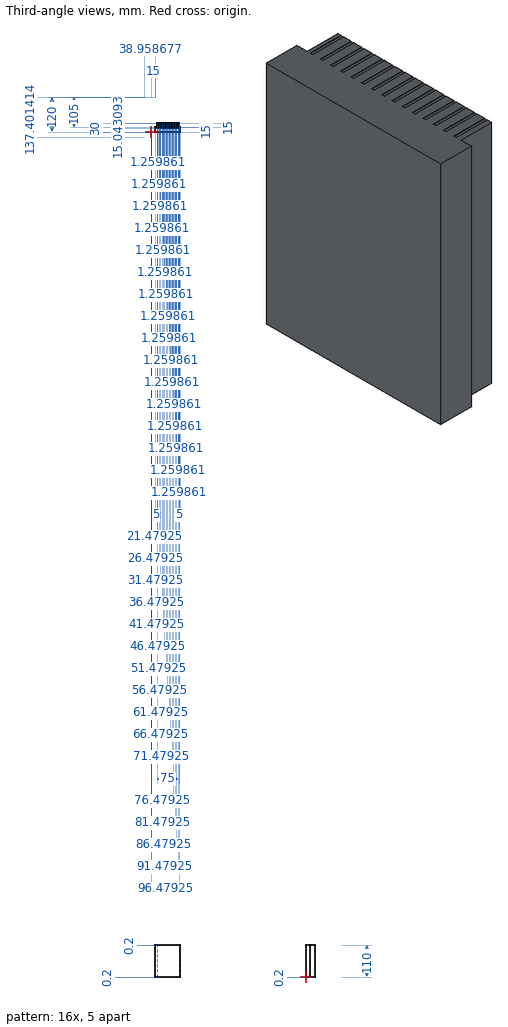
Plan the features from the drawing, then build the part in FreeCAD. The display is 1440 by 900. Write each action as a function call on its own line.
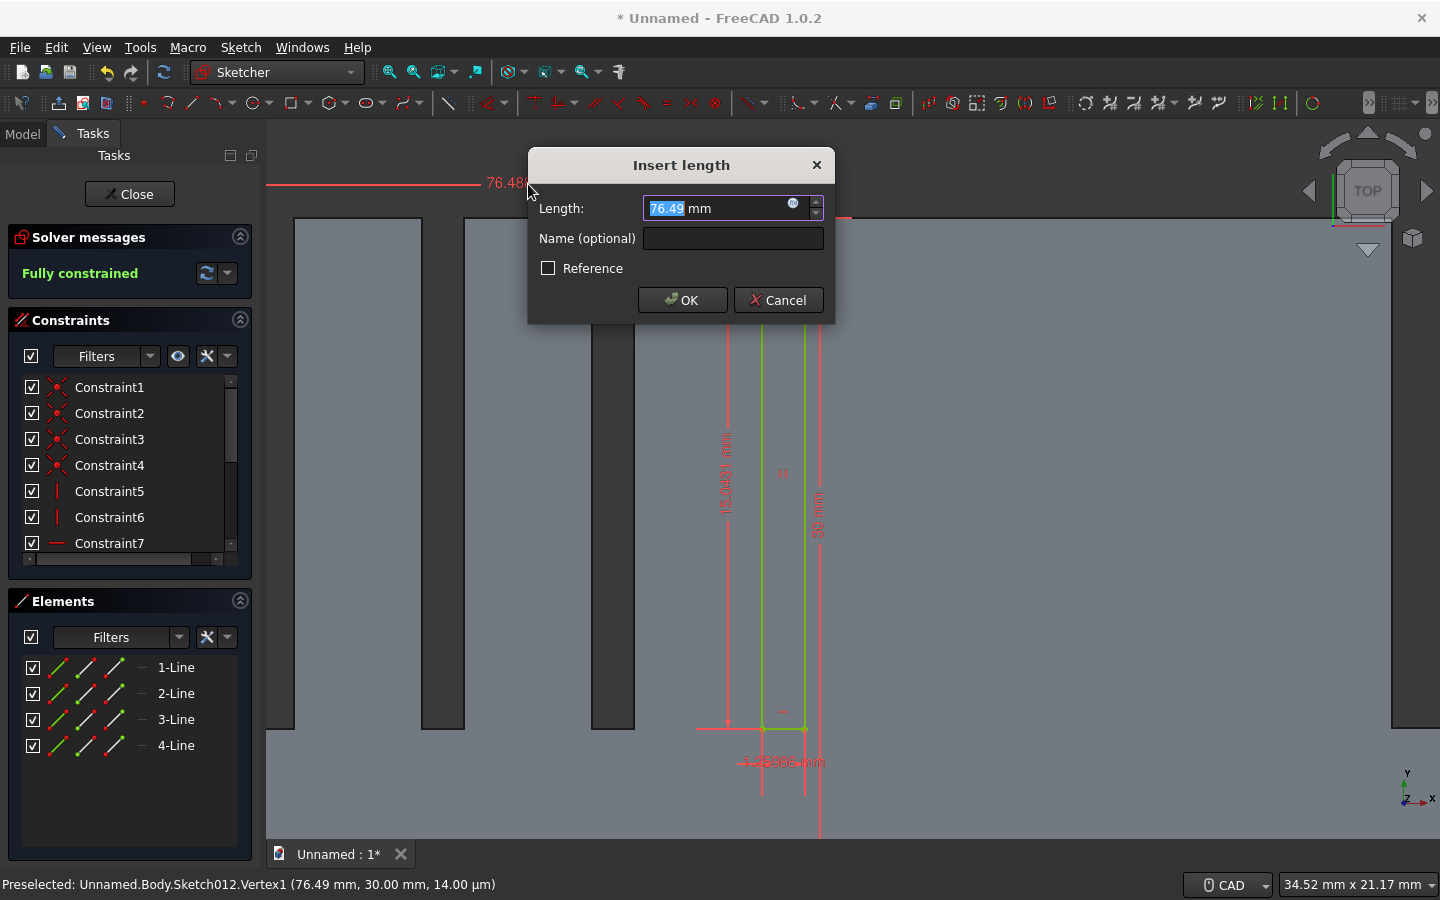
text(76.47925)
key(Return)
key(Escape)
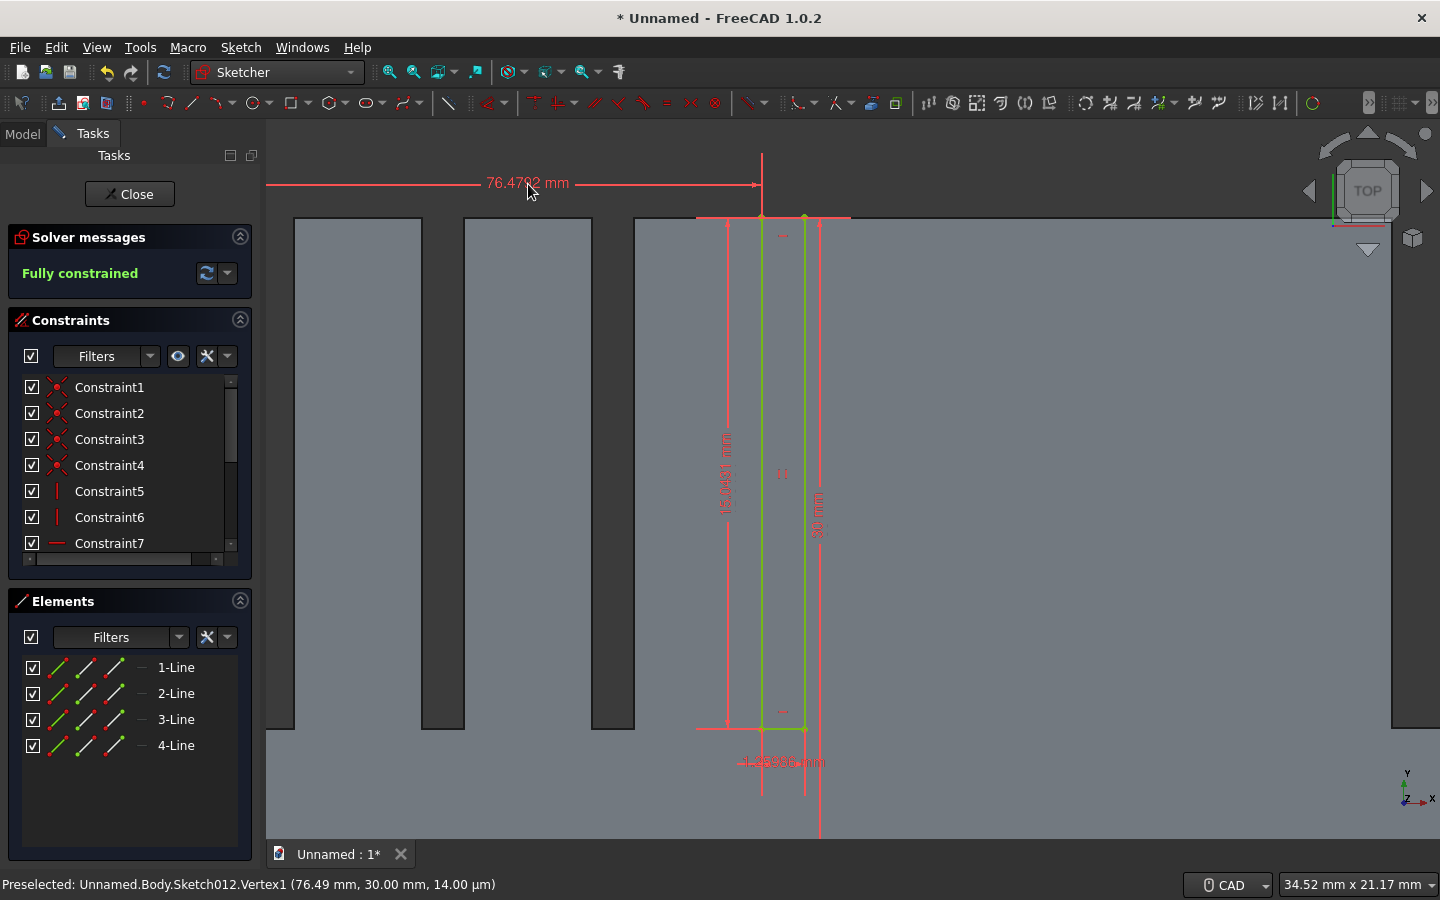
click(130, 194)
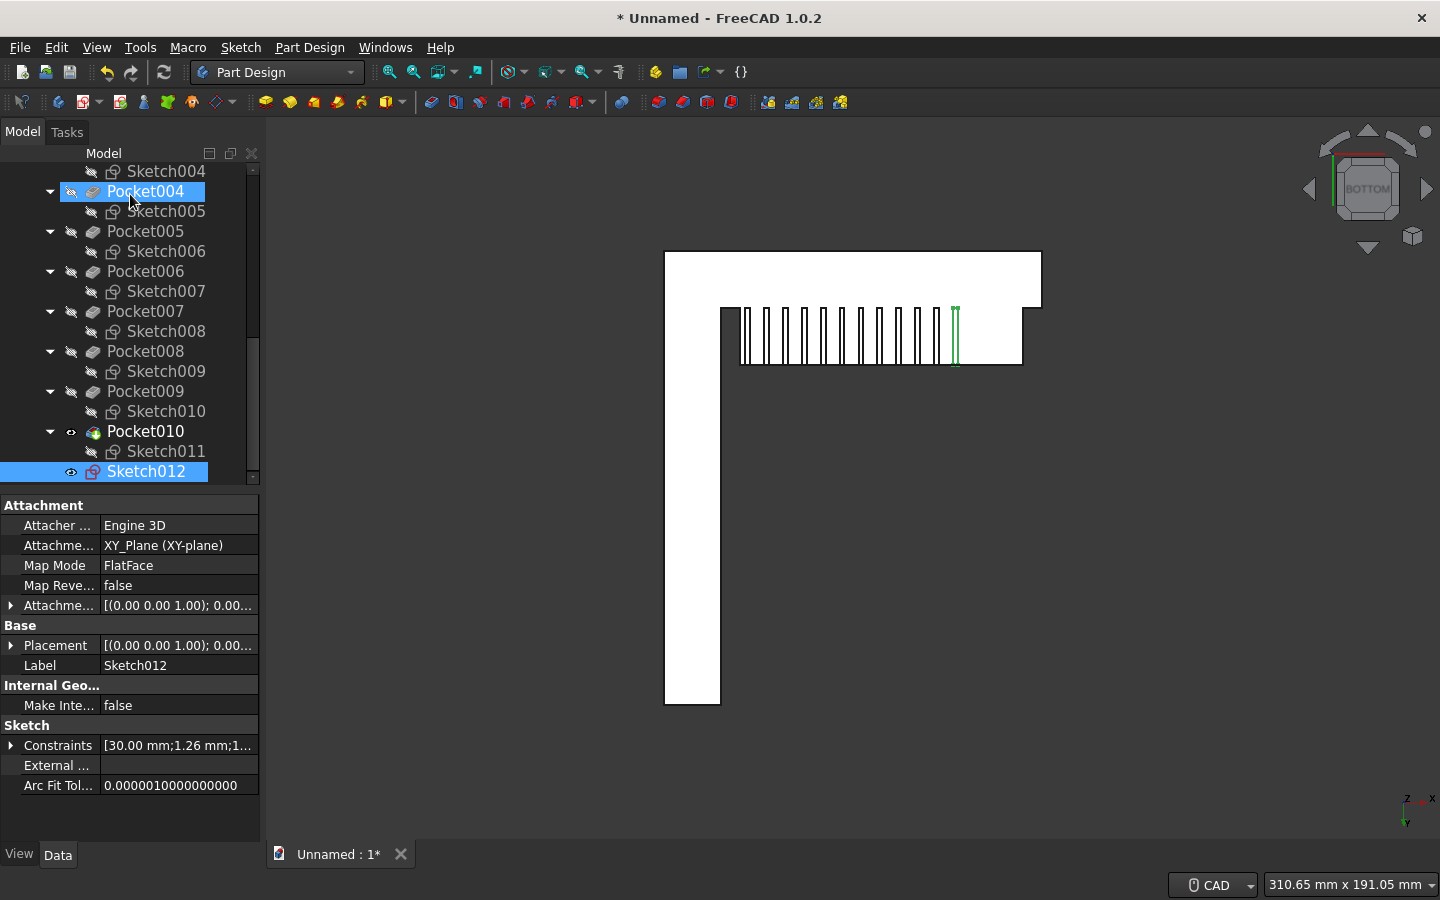
click(432, 102)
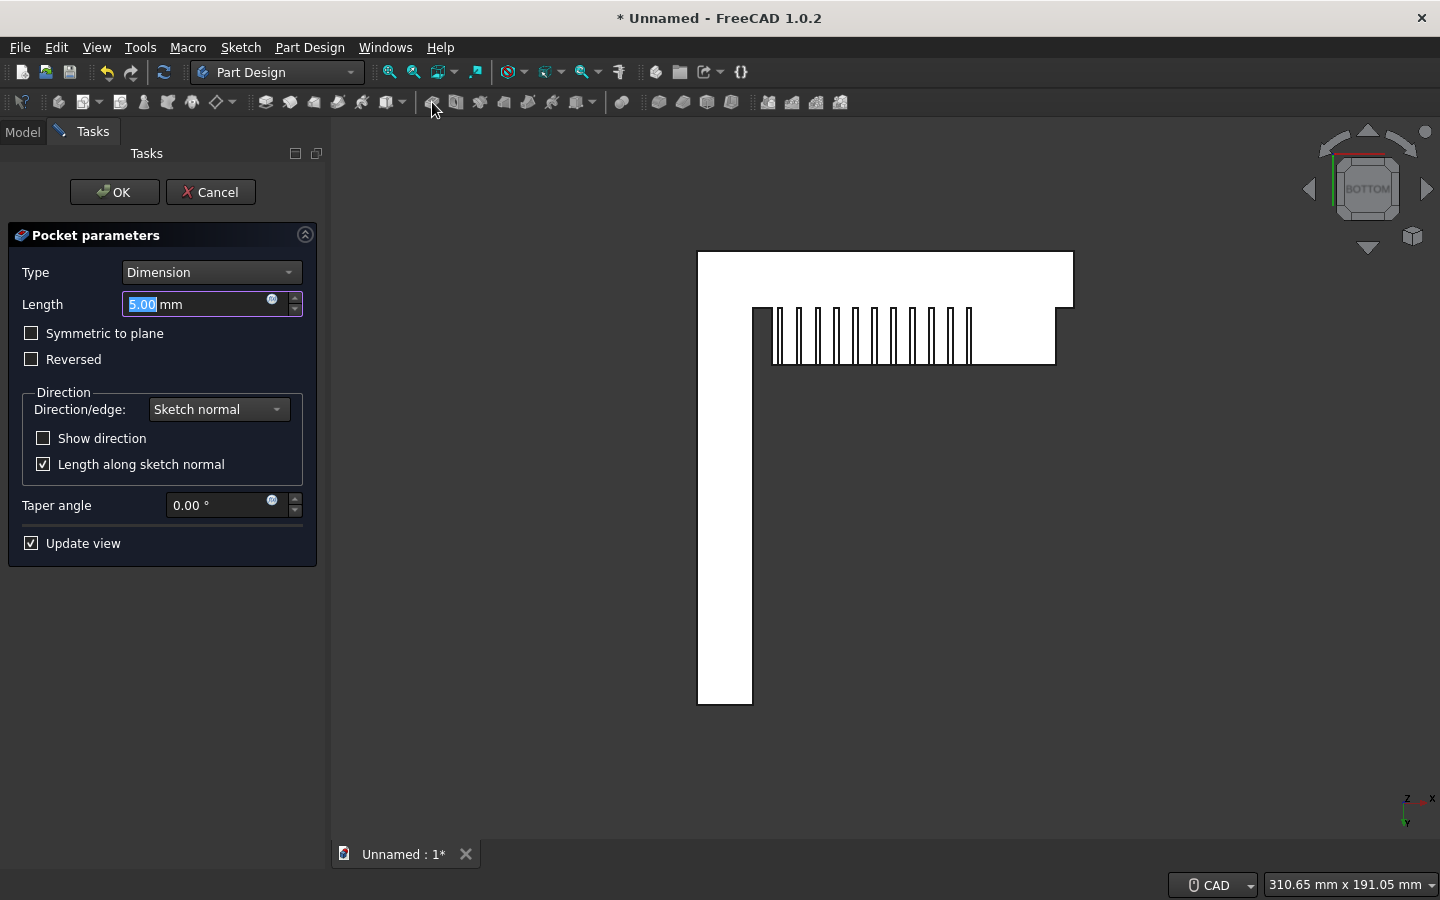
text(0.2)
key(Tab)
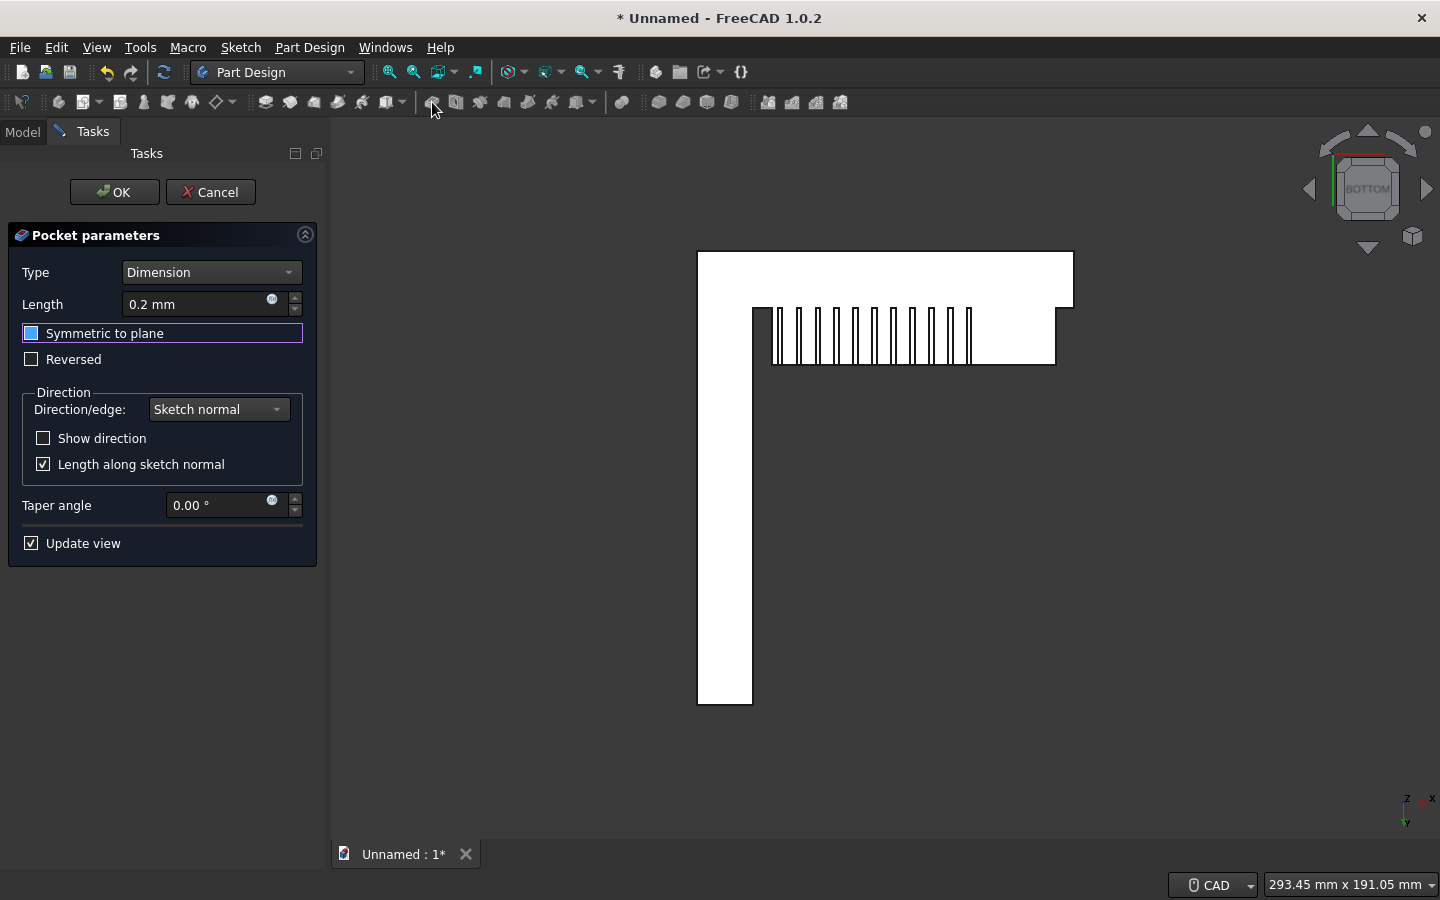
click(30, 359)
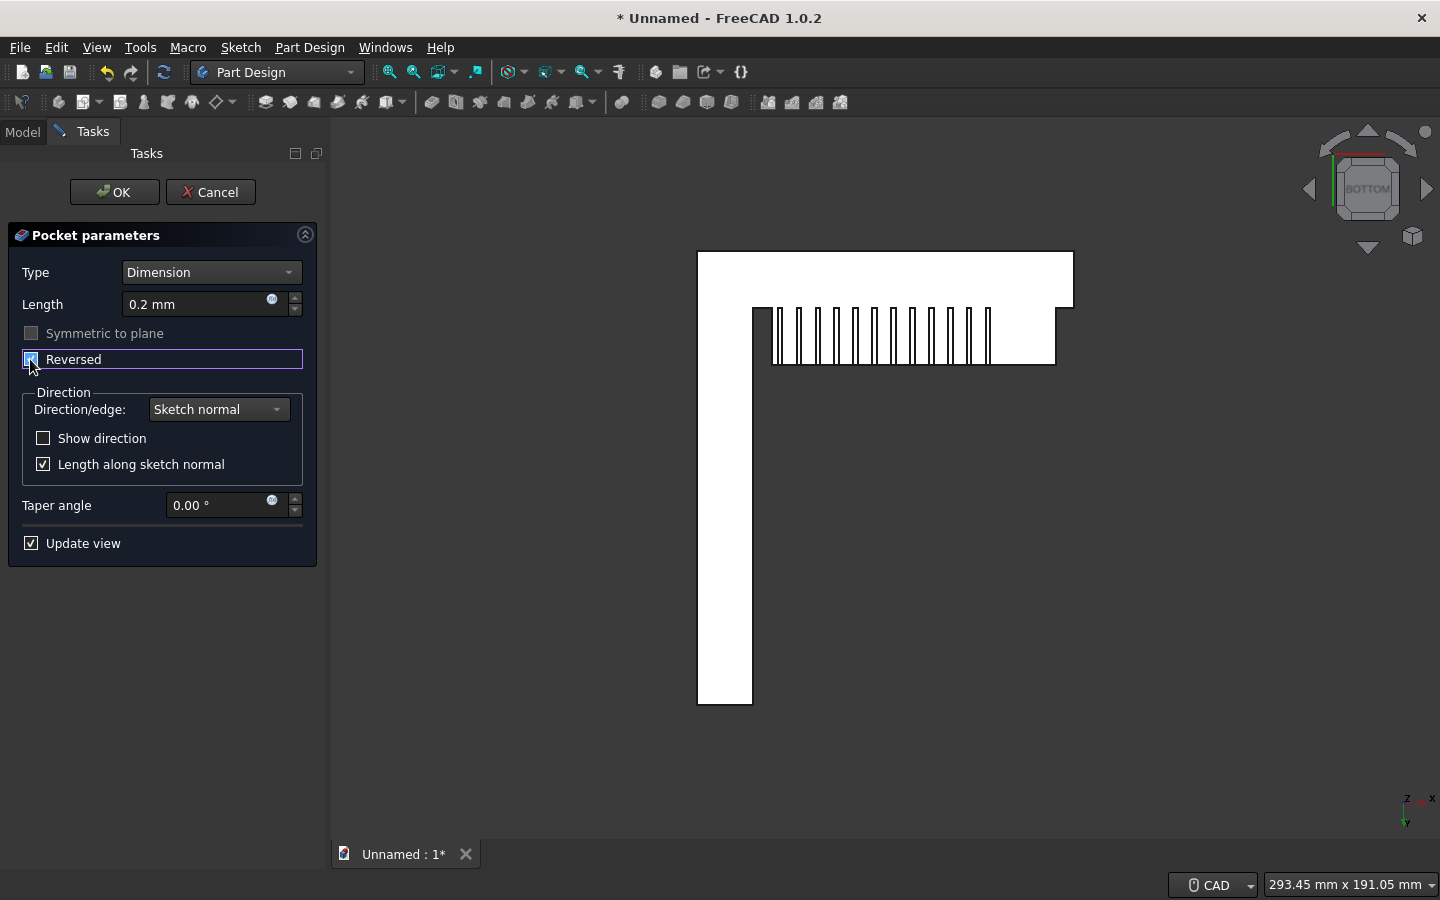
click(115, 192)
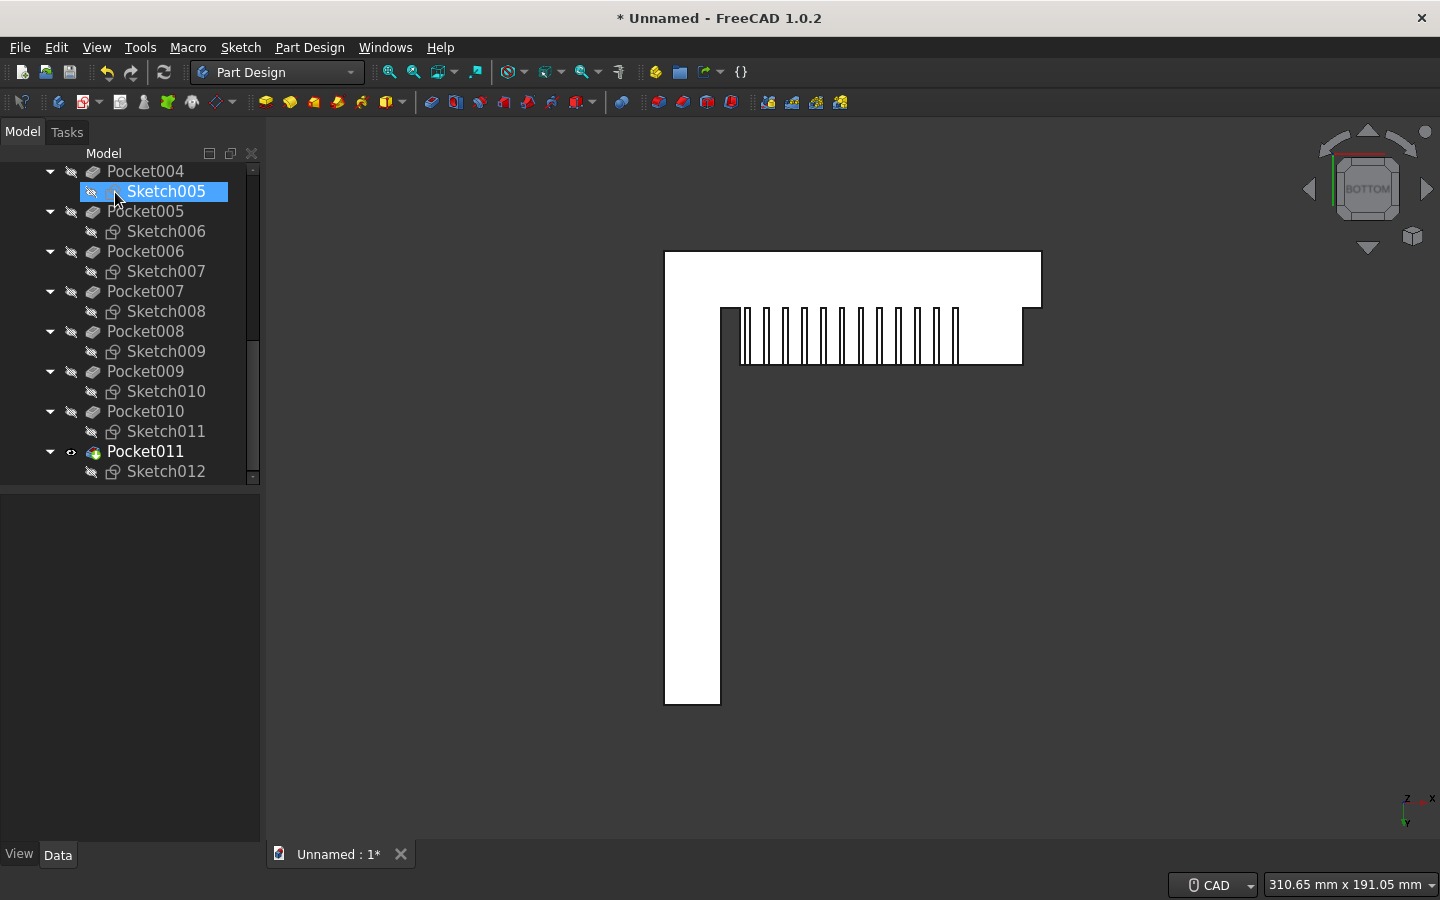
click(691, 671)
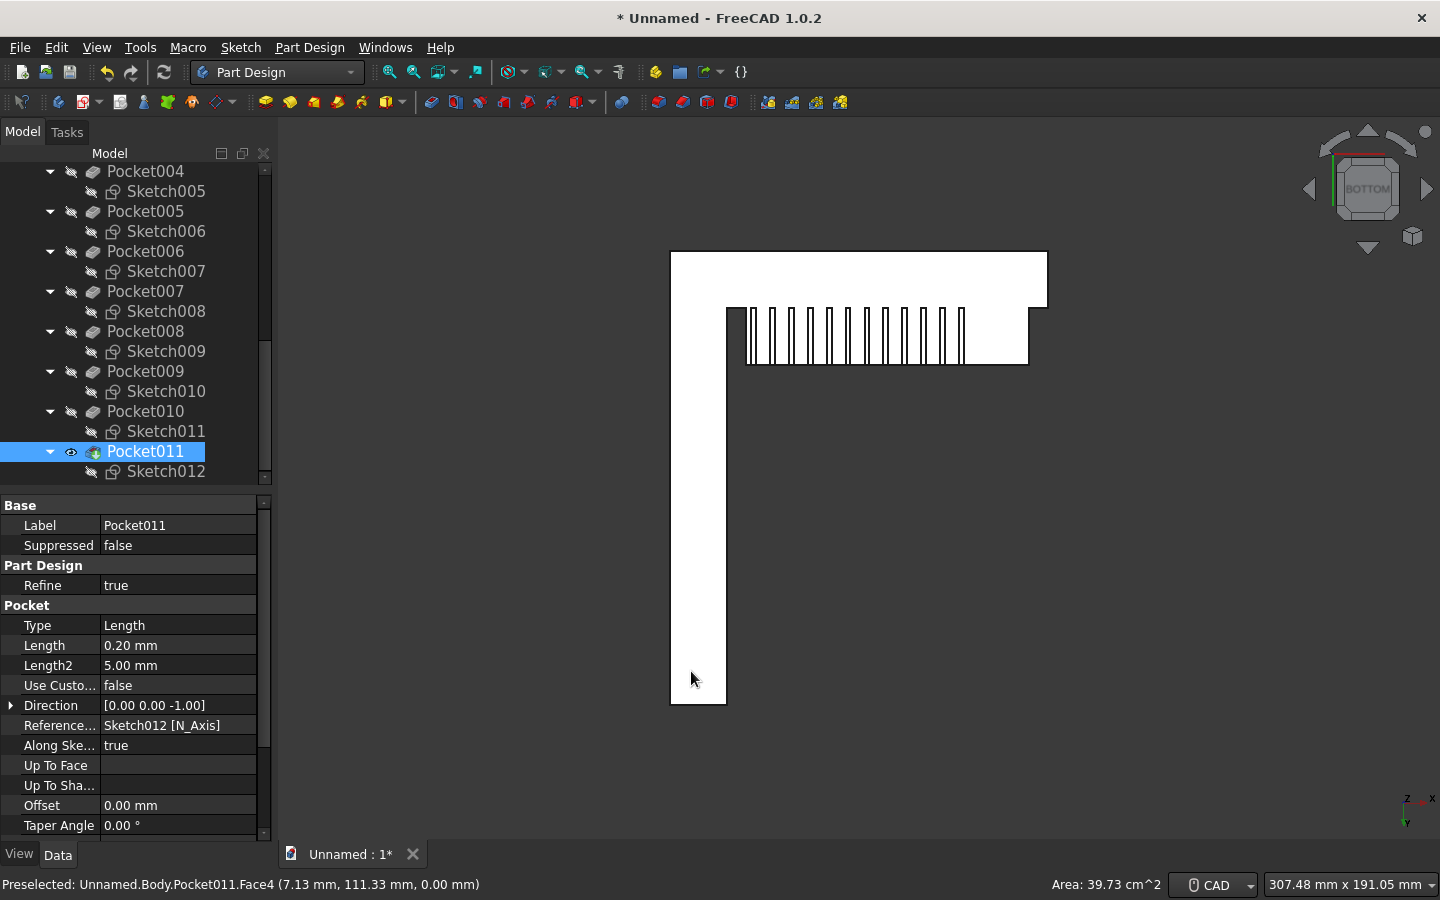
click(84, 102)